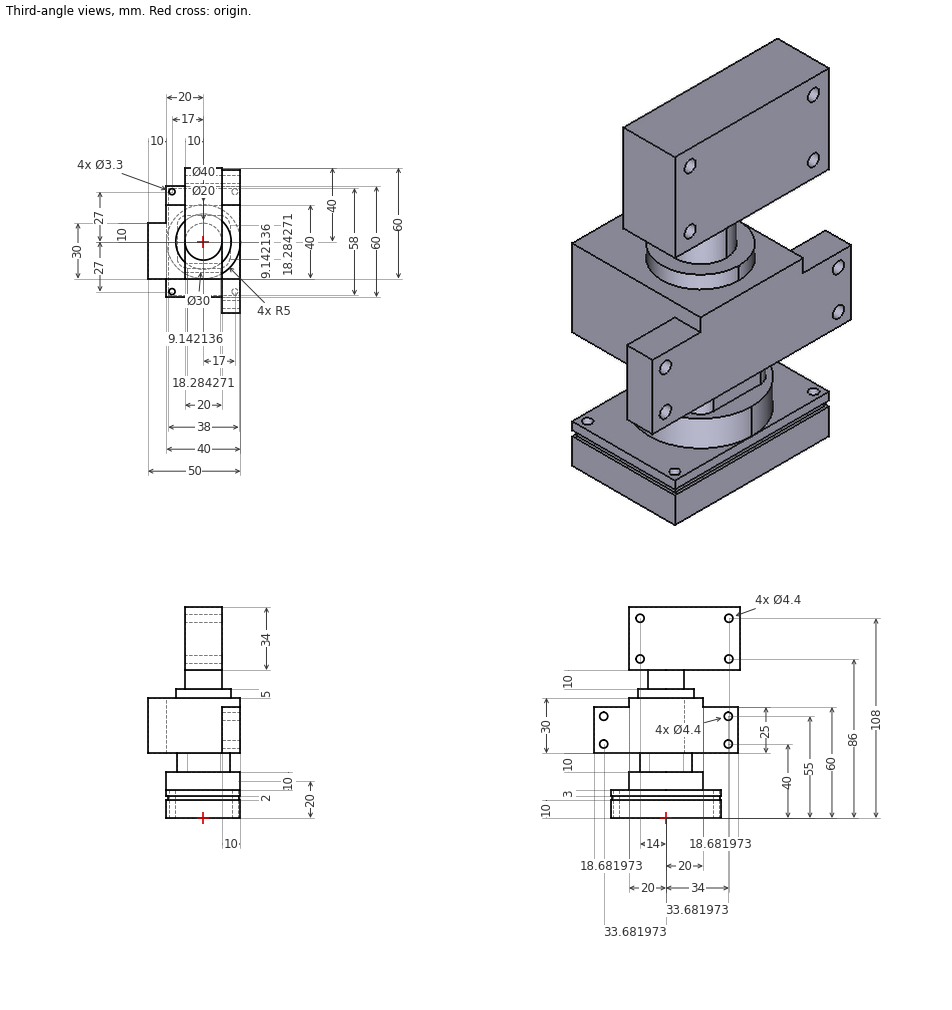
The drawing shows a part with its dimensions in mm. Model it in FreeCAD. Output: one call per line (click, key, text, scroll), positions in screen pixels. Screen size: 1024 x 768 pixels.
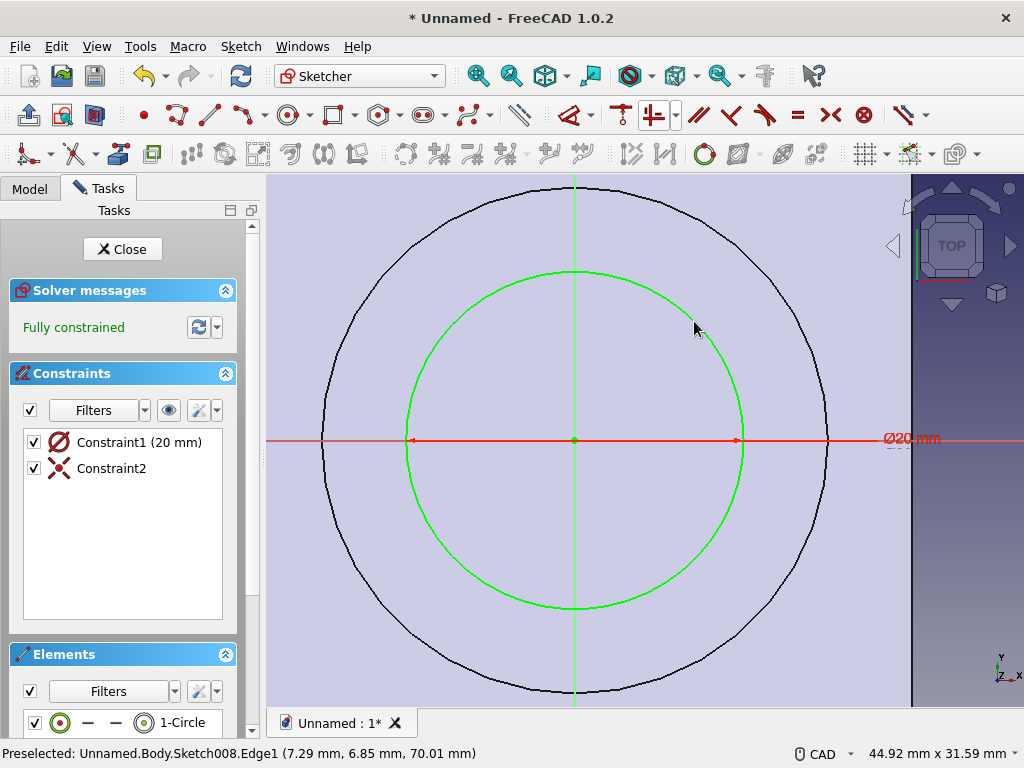
click(123, 249)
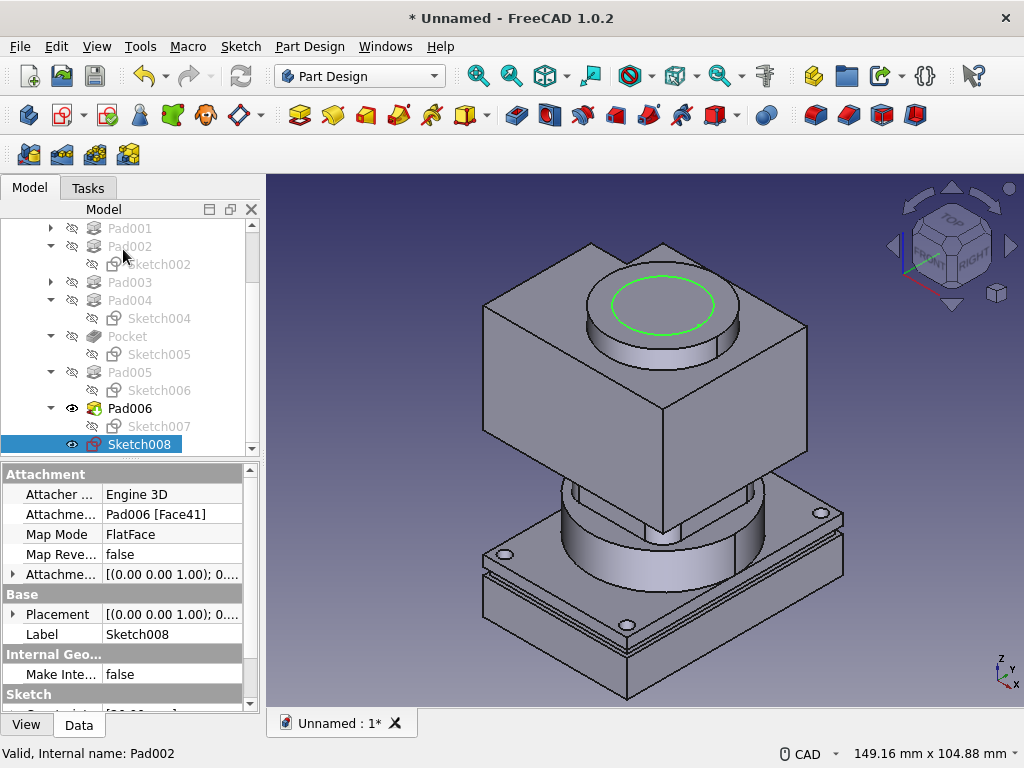
click(300, 116)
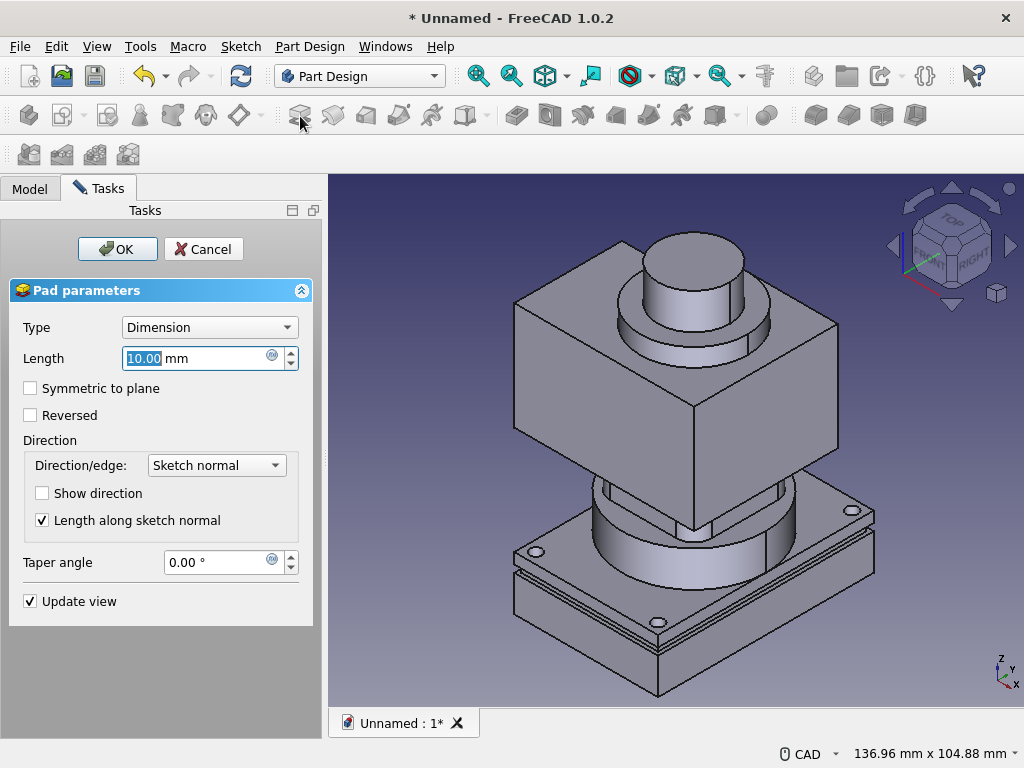
text(10)
key(Tab)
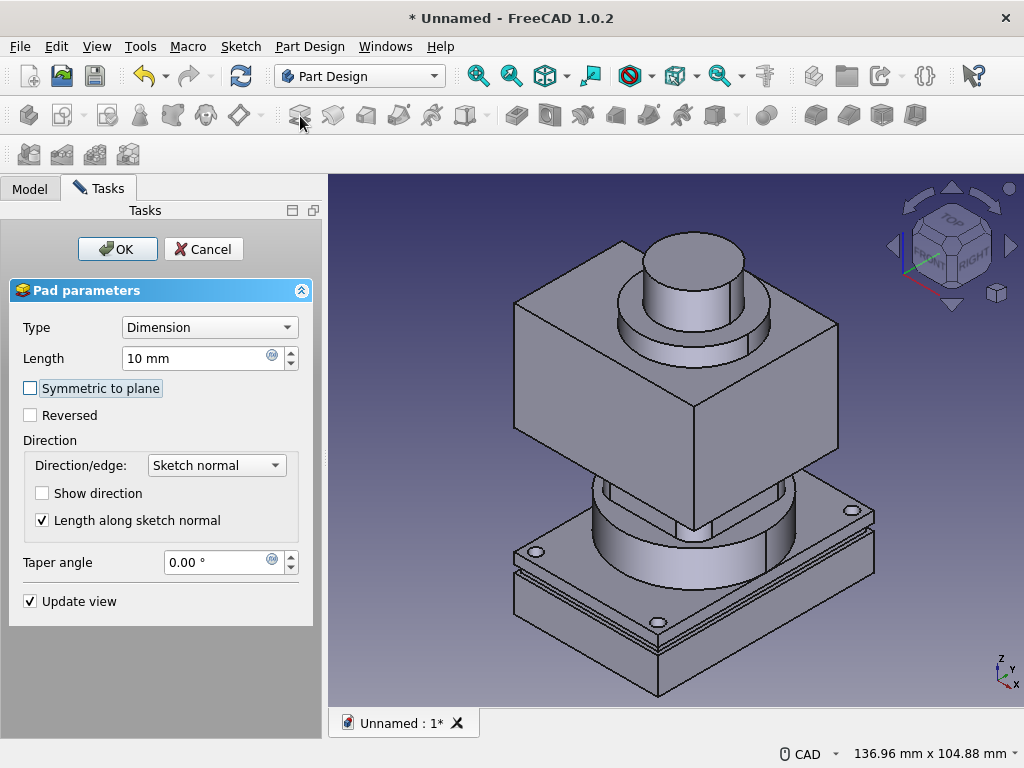
click(118, 249)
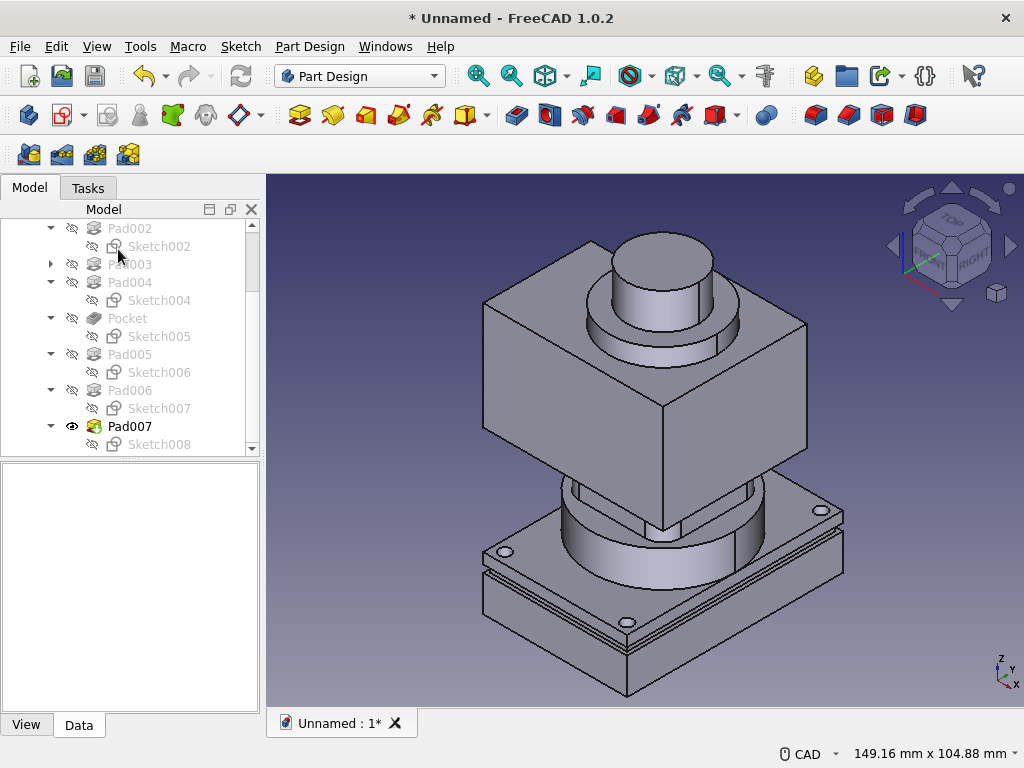
click(479, 76)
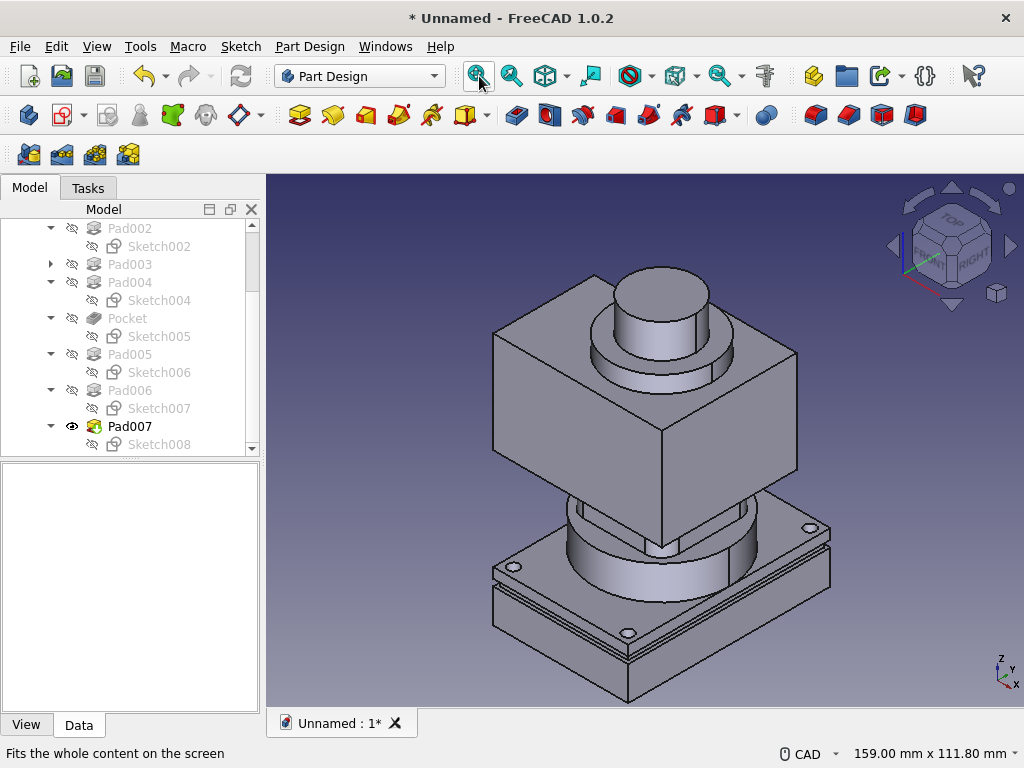
click(729, 449)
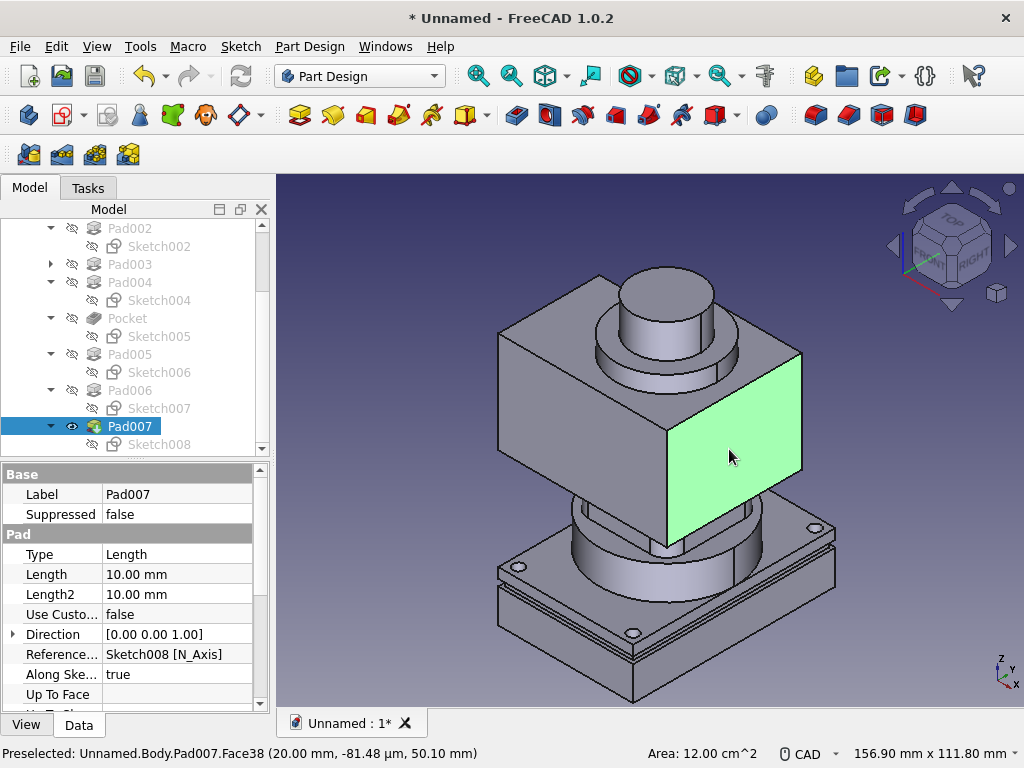
click(62, 116)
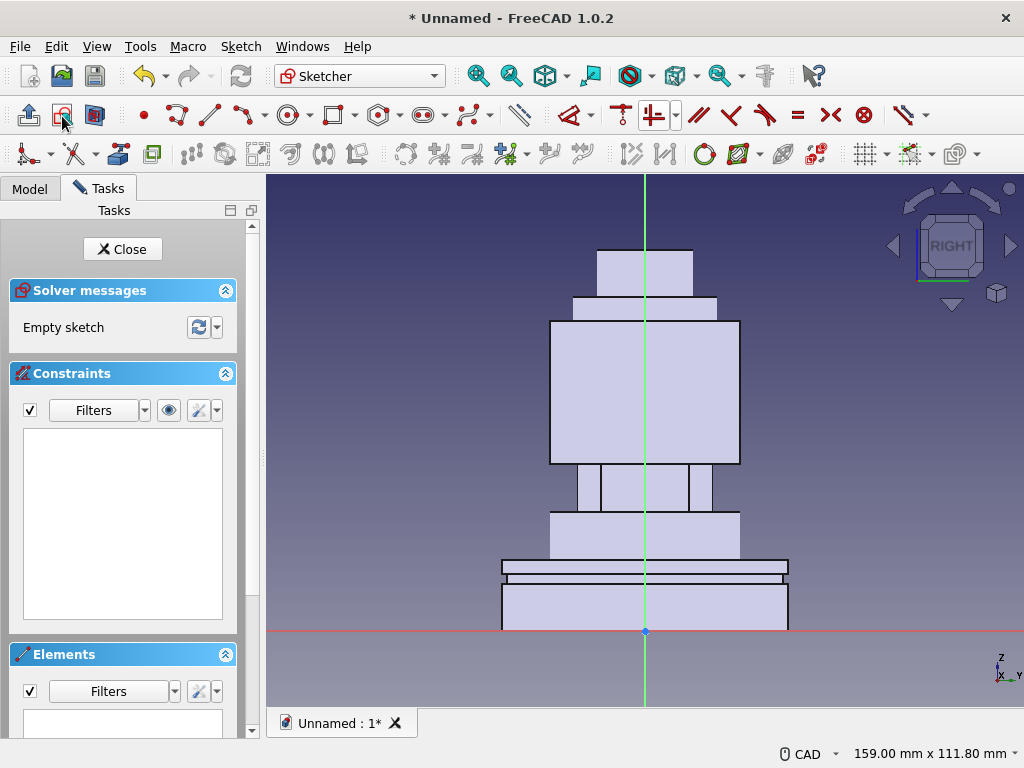
key(g)
key(r)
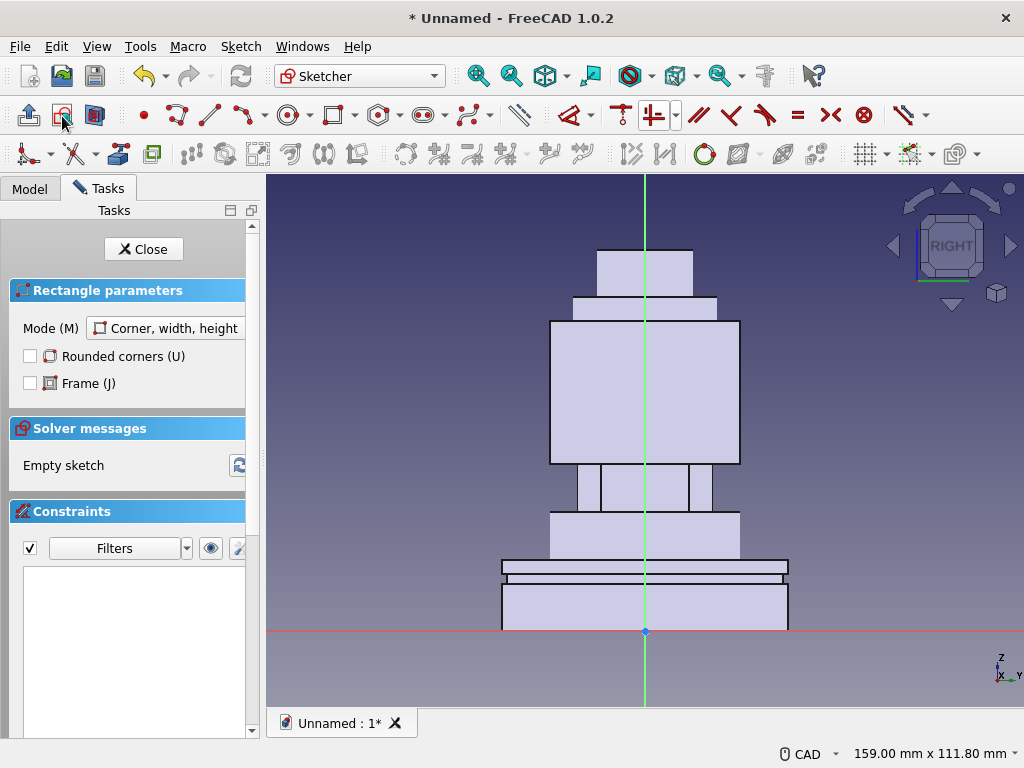
click(740, 345)
move(829, 464)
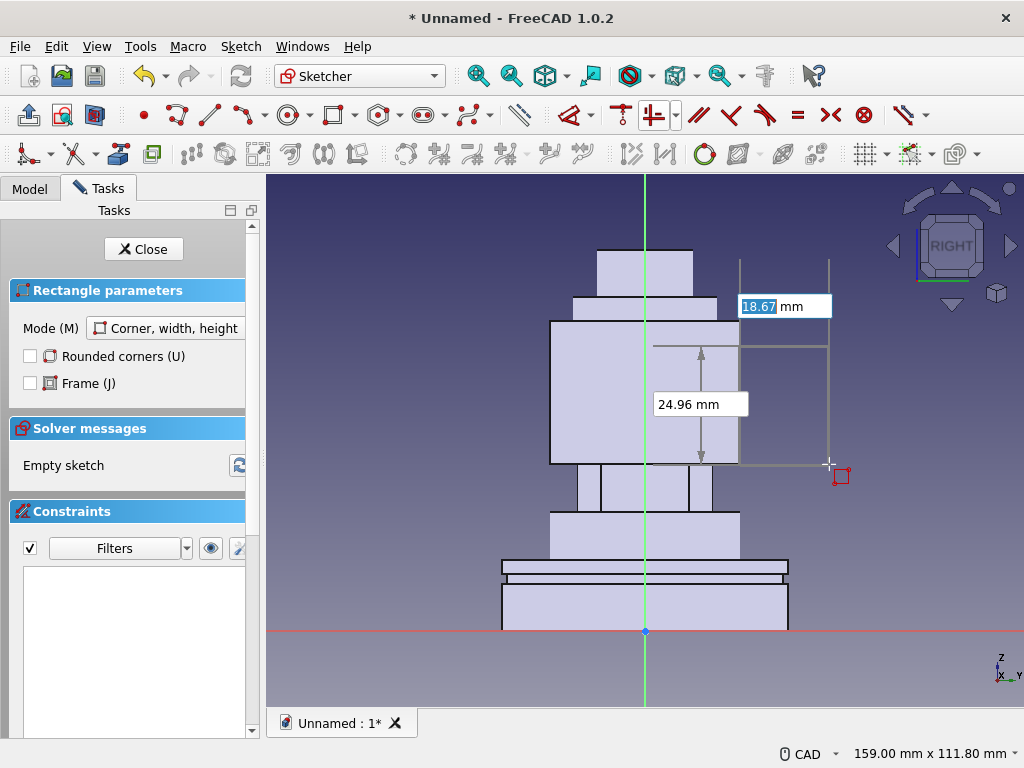
text(18.681973)
key(Tab)
text(25)
key(Return)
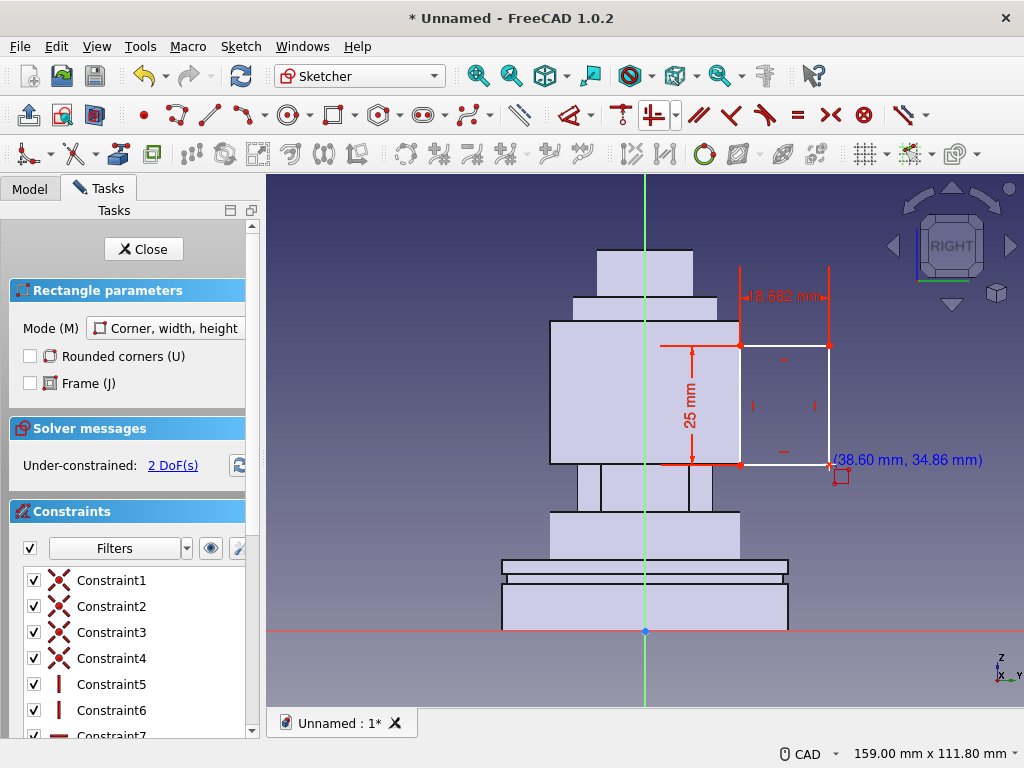
click(461, 345)
move(550, 464)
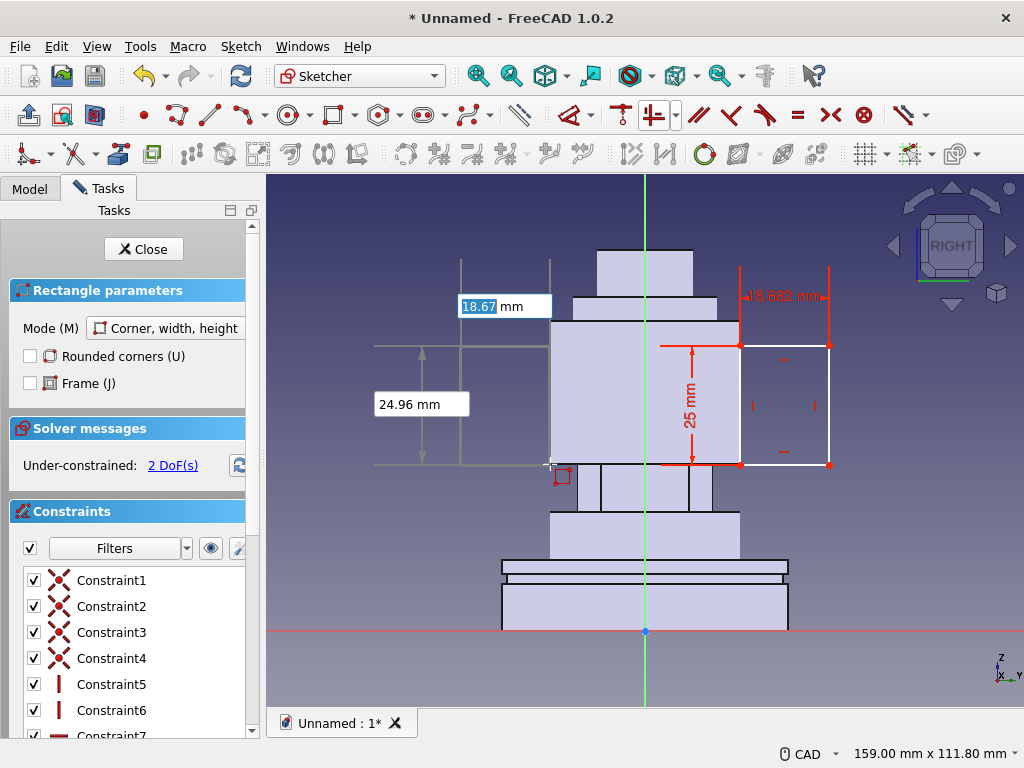
text(18.681973)
key(Tab)
text(25)
key(Return)
key(Escape)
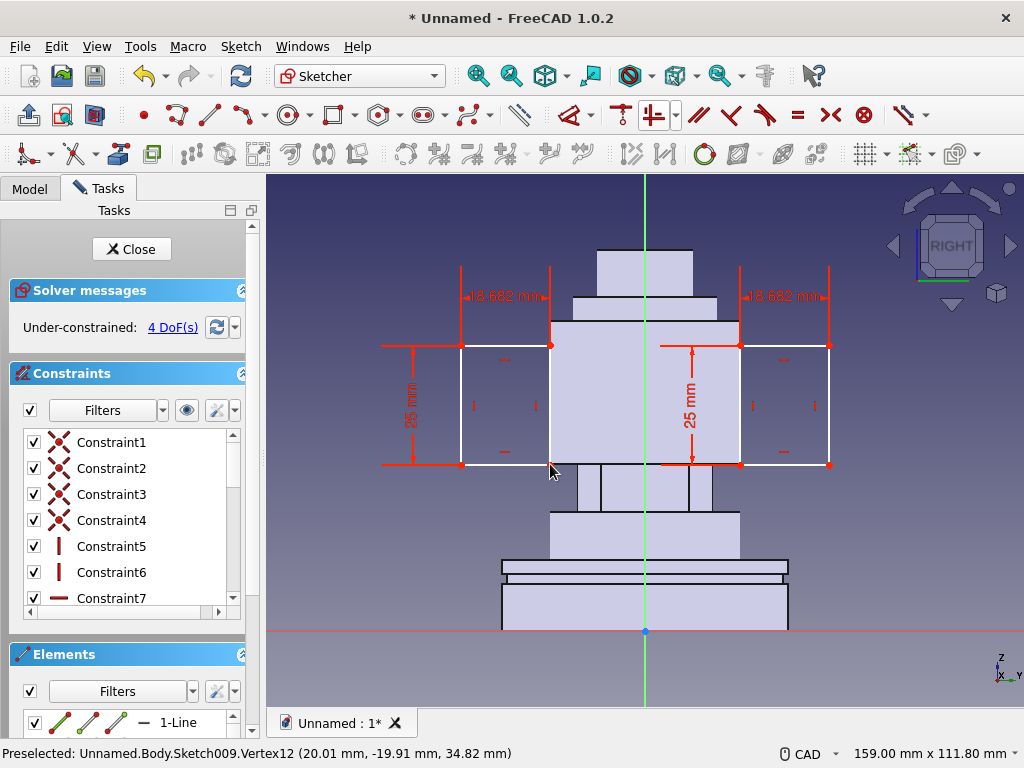
click(568, 116)